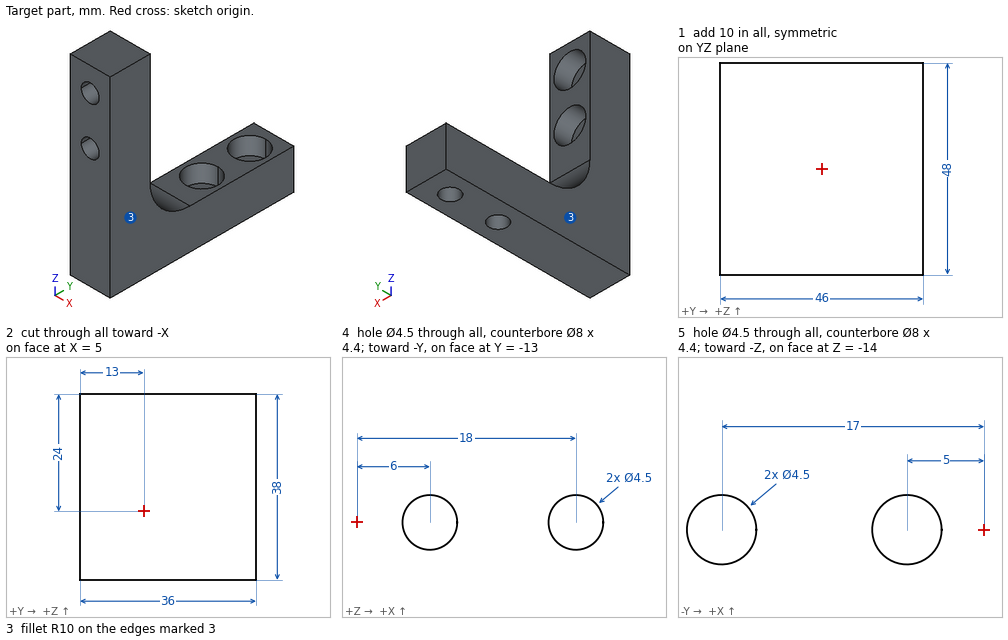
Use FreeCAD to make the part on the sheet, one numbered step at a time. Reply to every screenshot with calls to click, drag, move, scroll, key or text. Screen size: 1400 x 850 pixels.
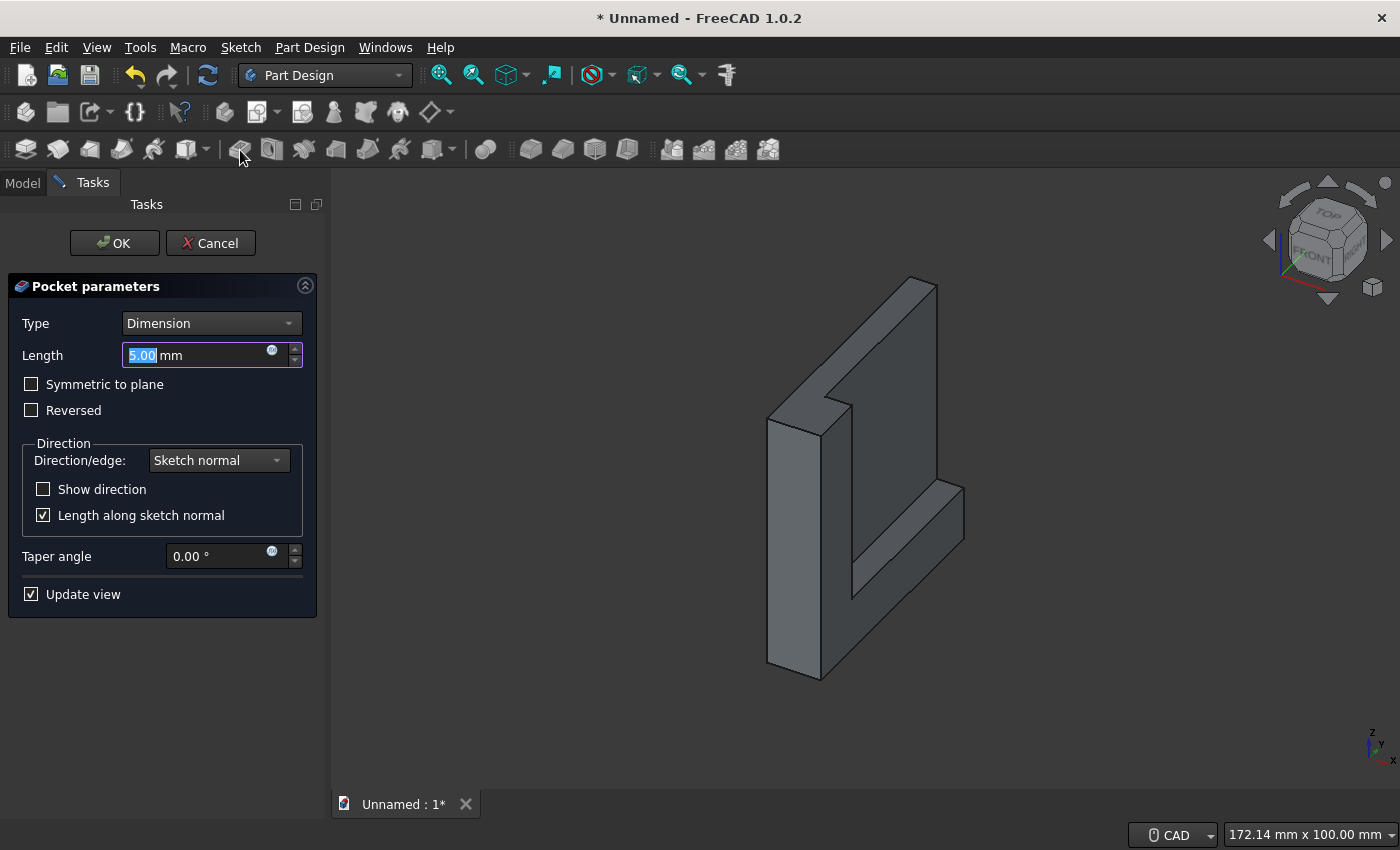
click(212, 324)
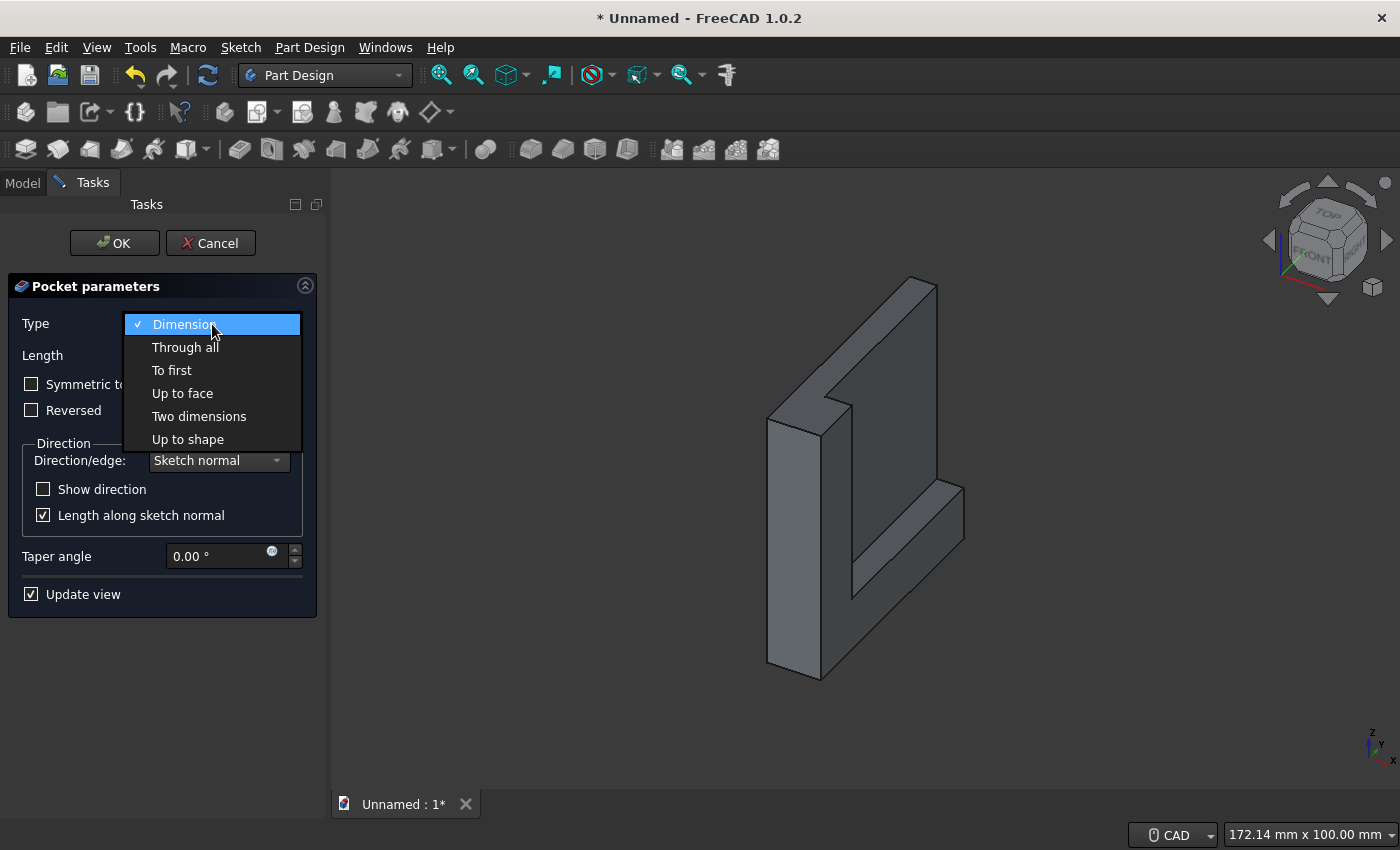
click(212, 348)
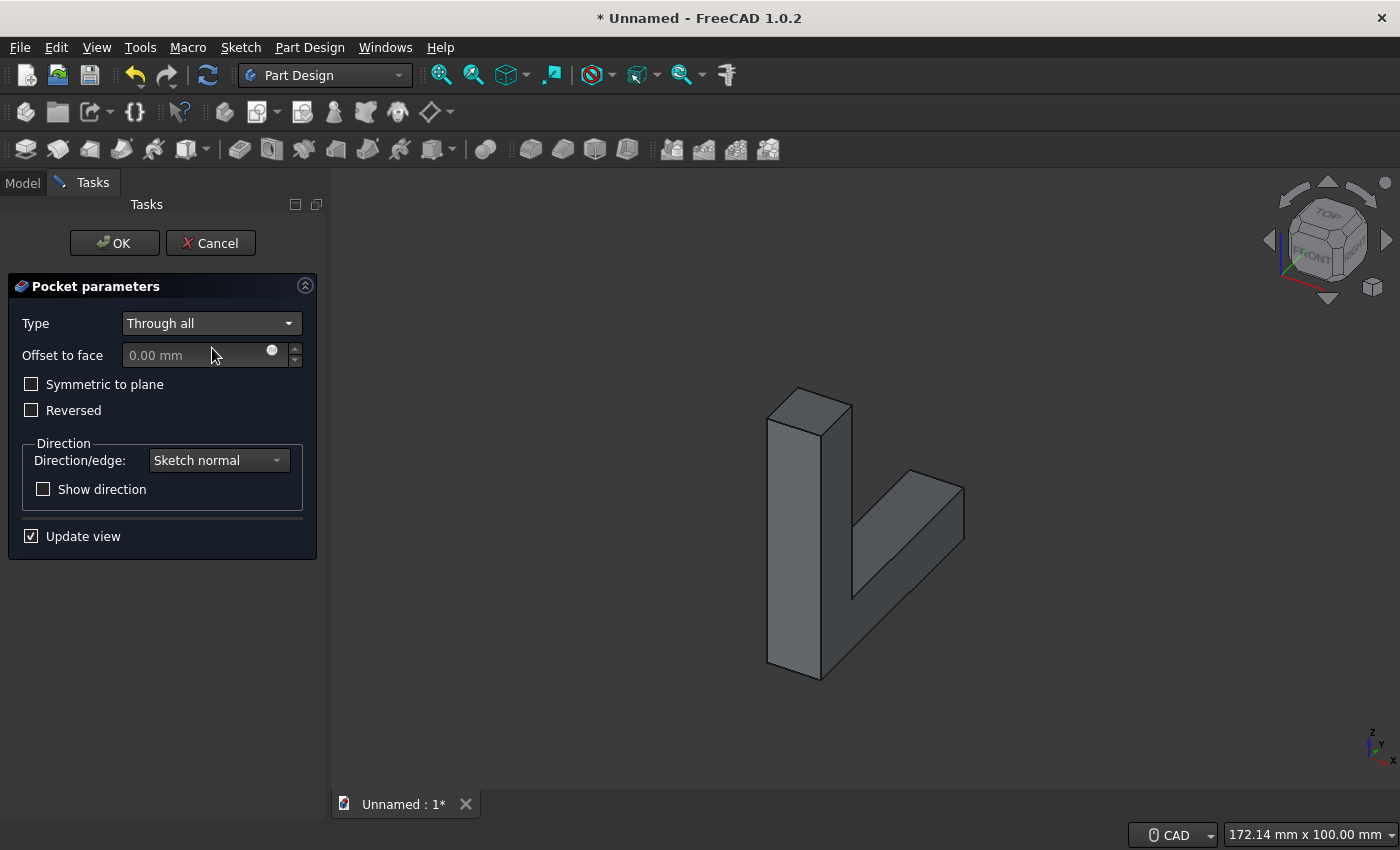
click(115, 243)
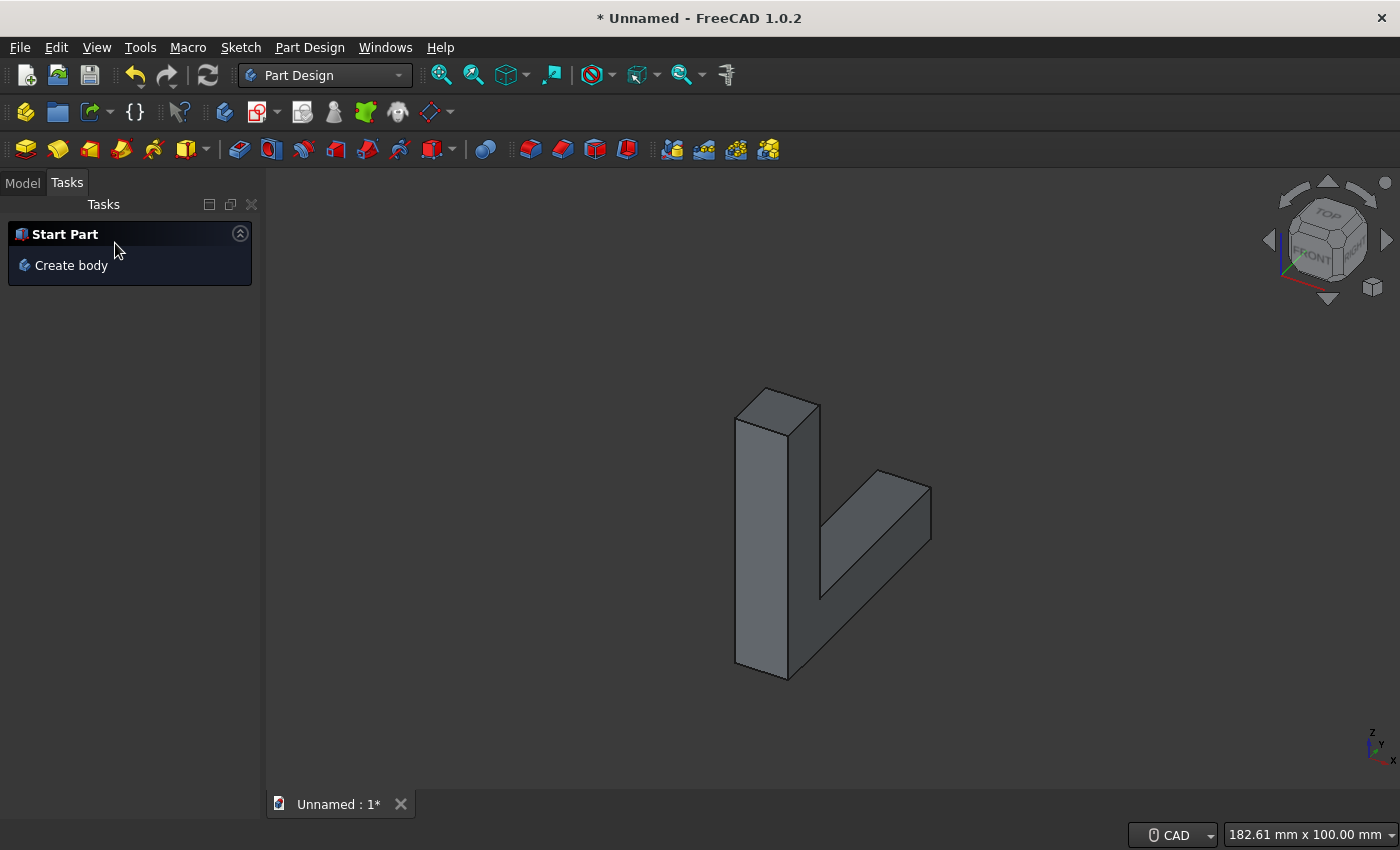
key(0)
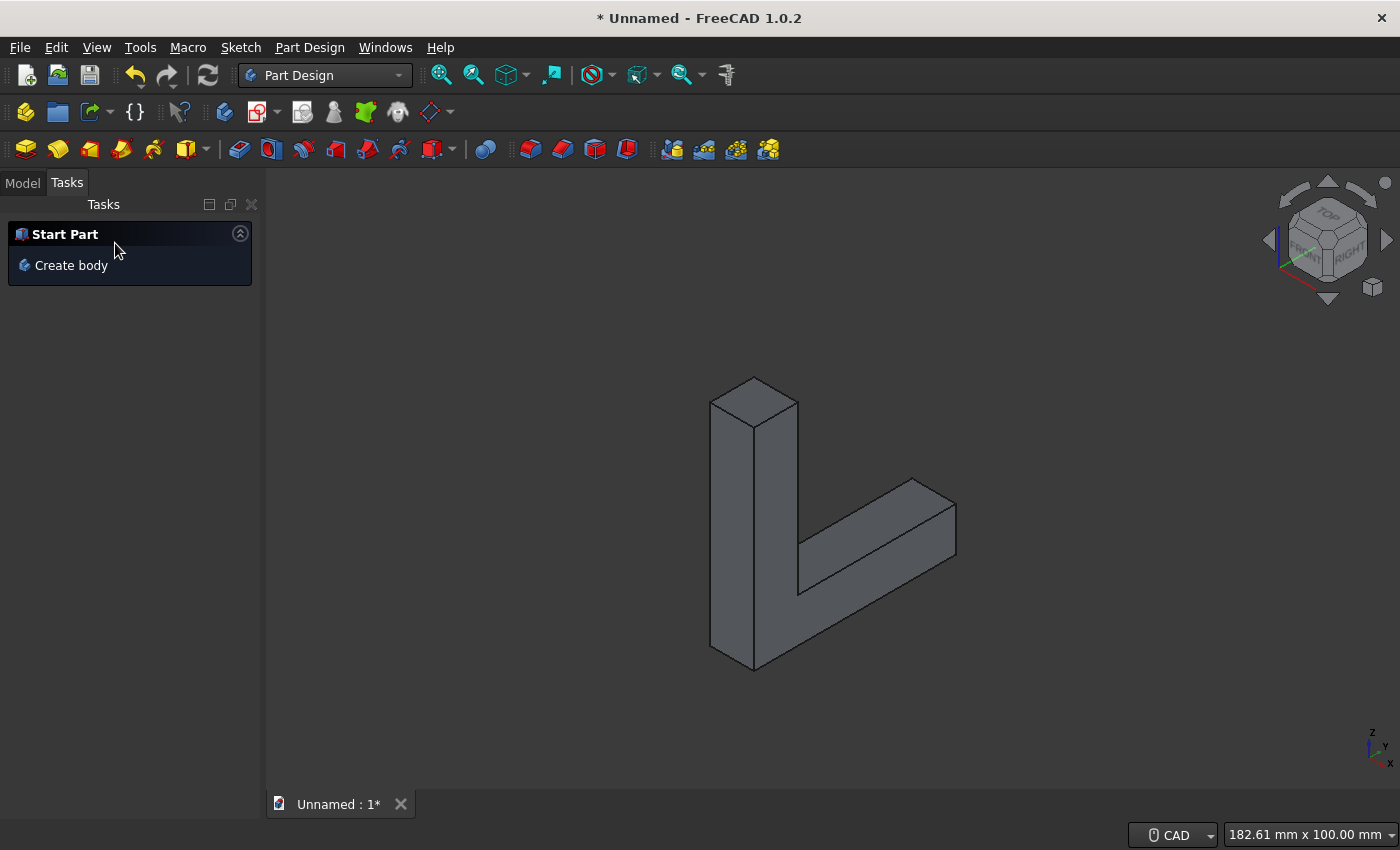
key(2)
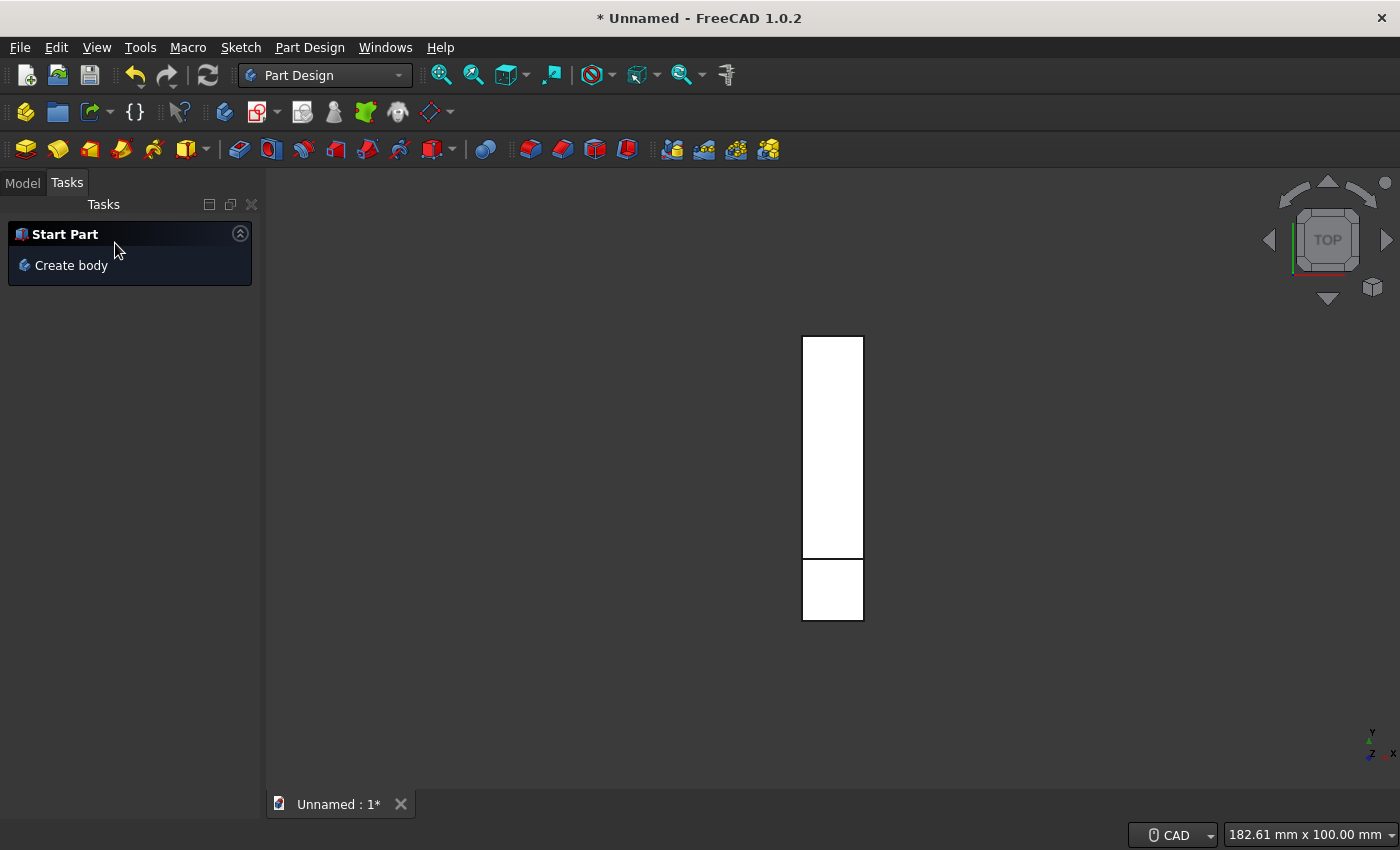
key(1)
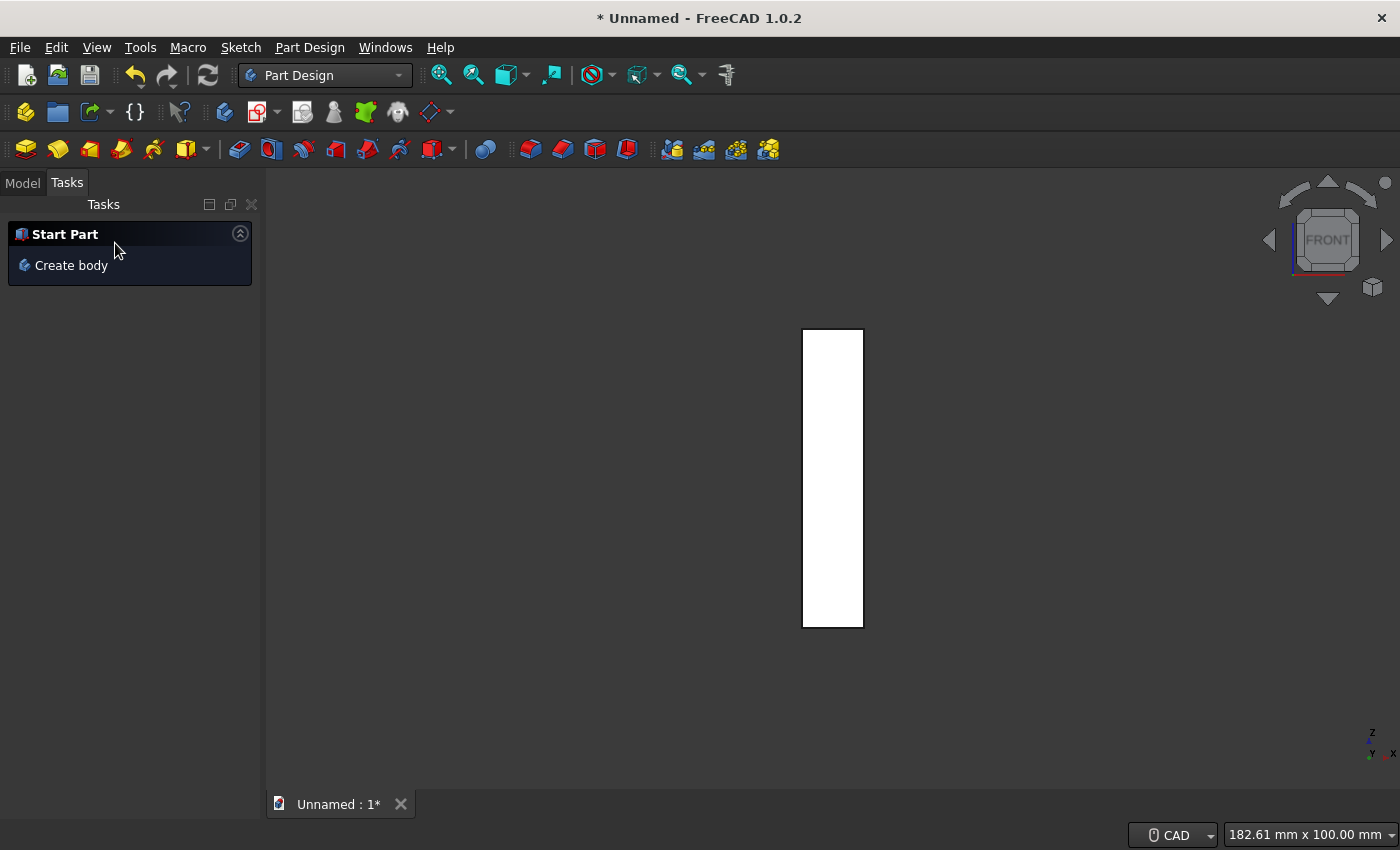
key(3)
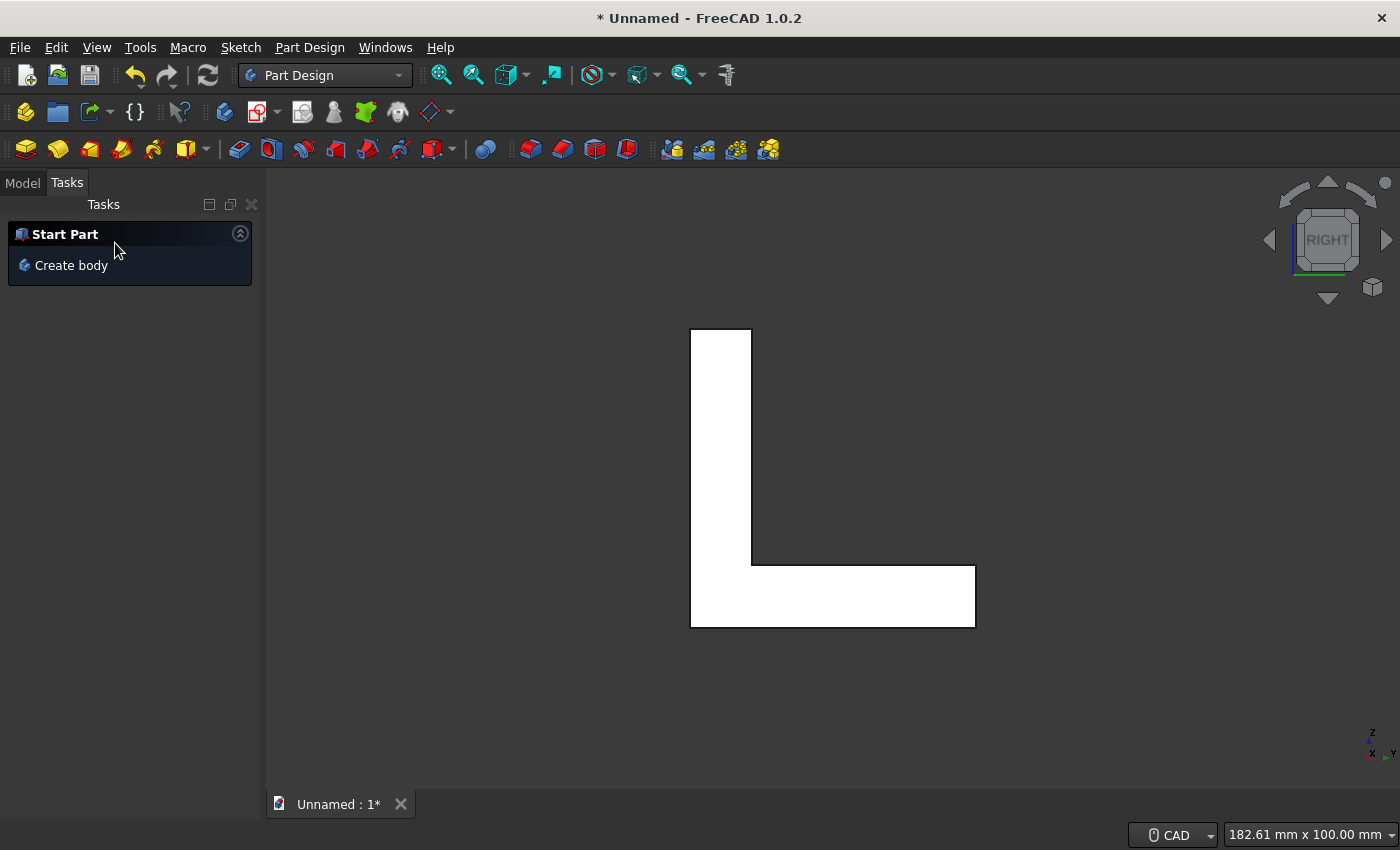
key(5)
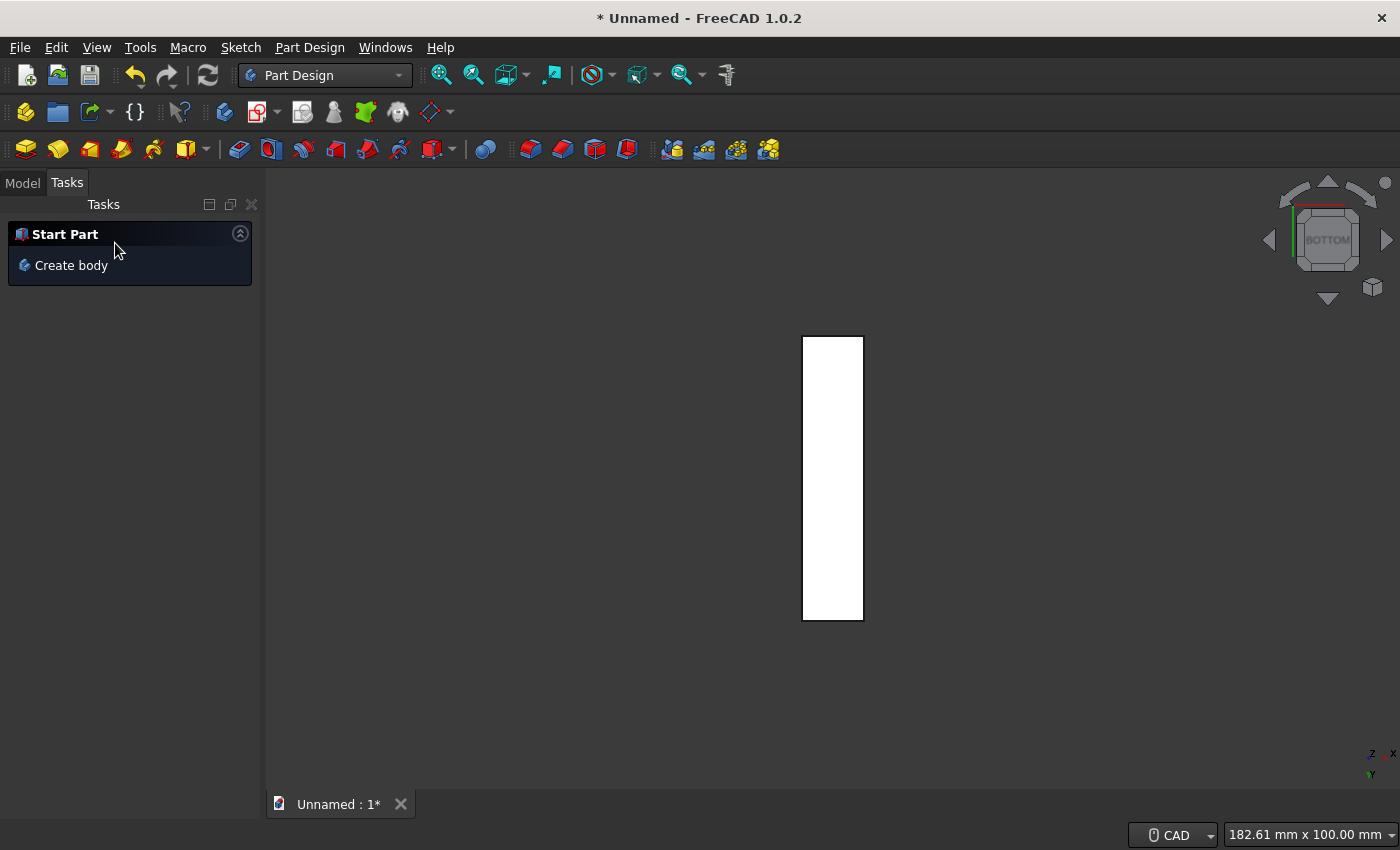
key(4)